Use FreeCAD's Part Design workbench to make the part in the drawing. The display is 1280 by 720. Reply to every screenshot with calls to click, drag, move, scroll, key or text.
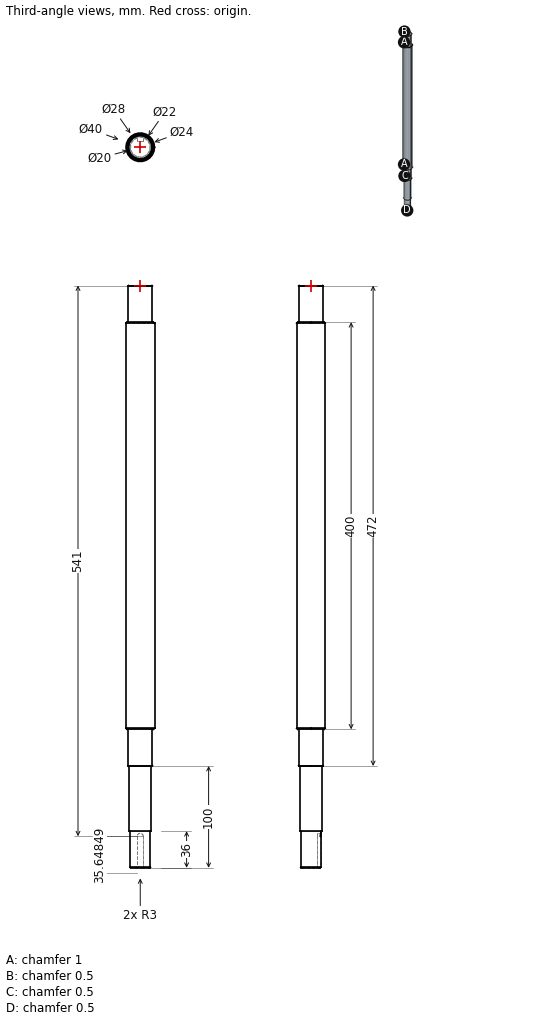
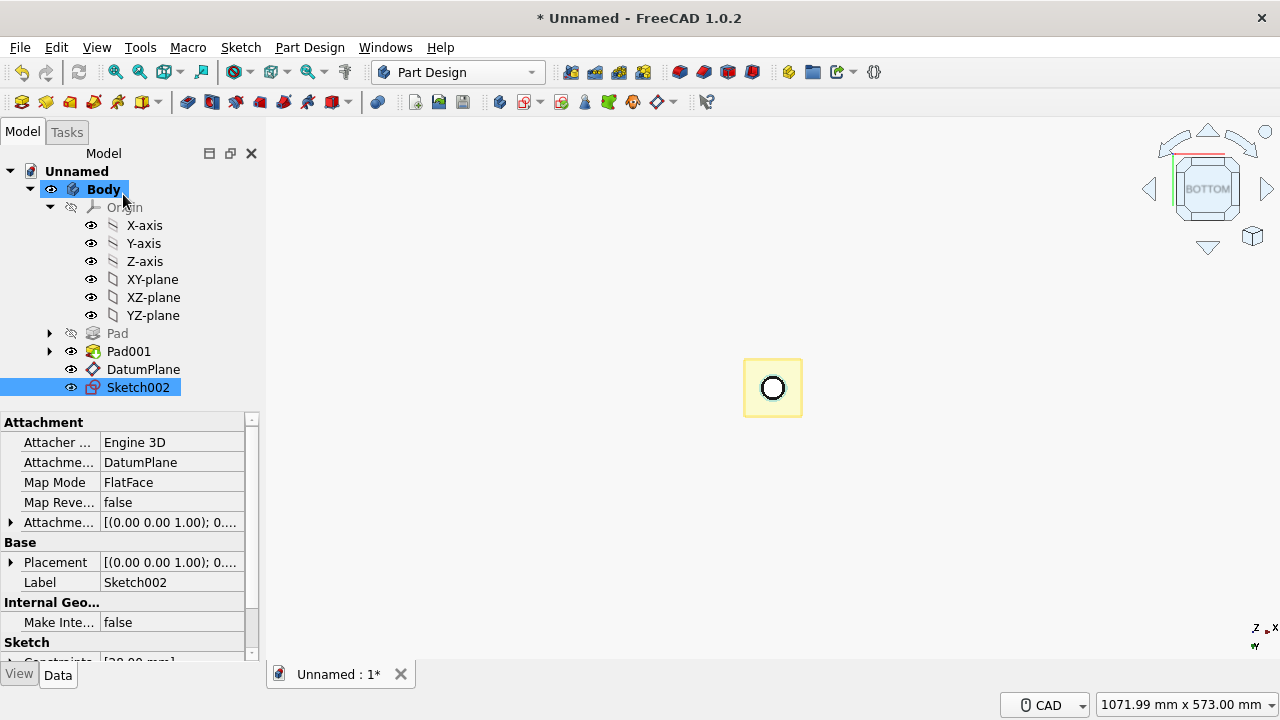
click(22, 102)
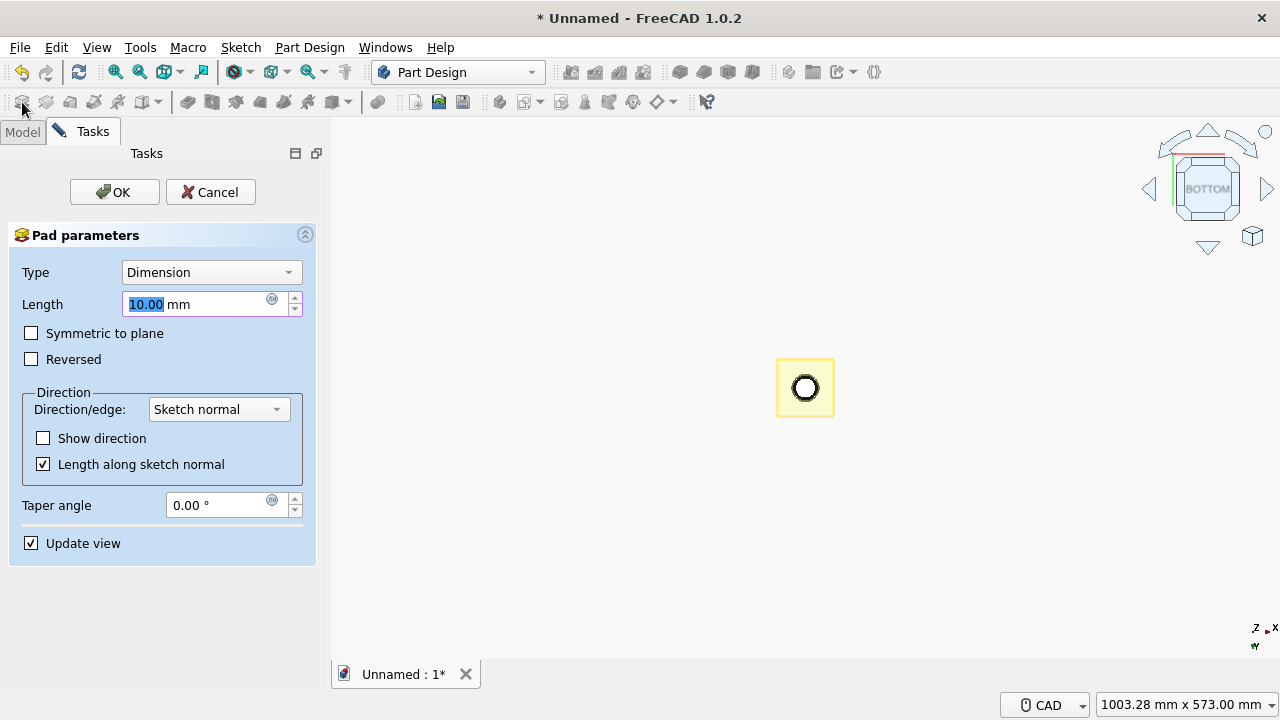
text(400)
key(Tab)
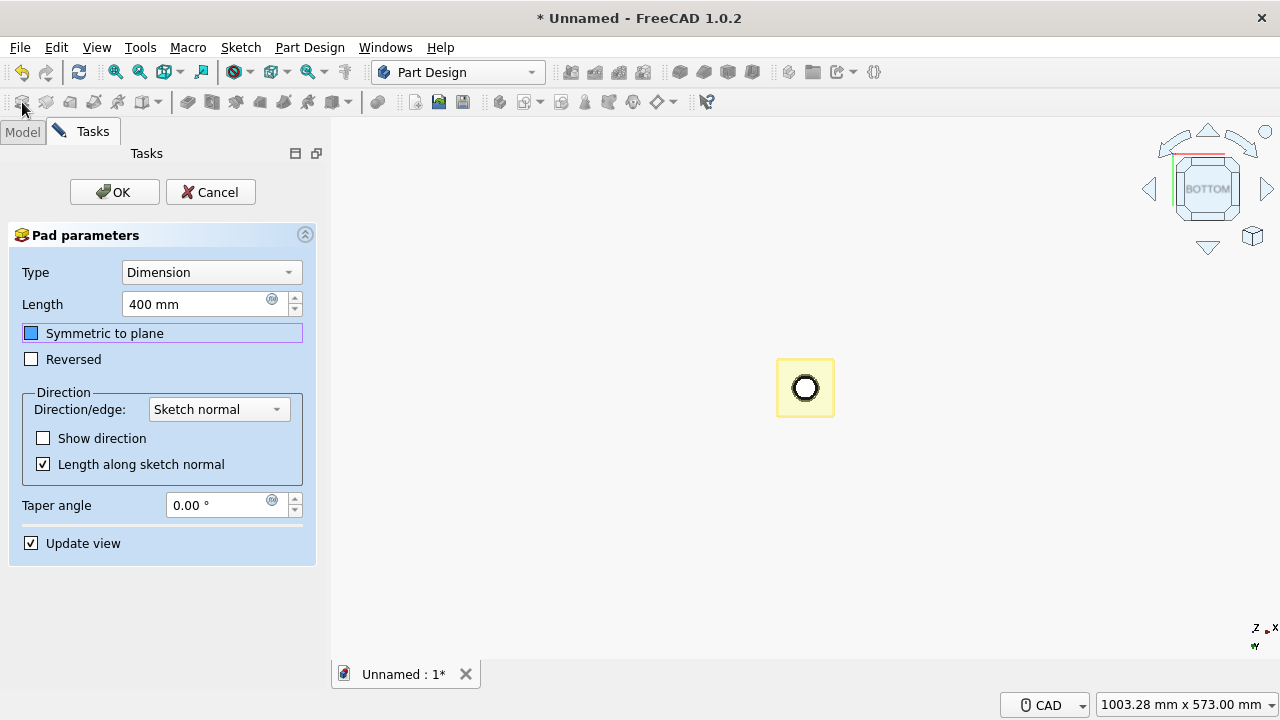
click(30, 359)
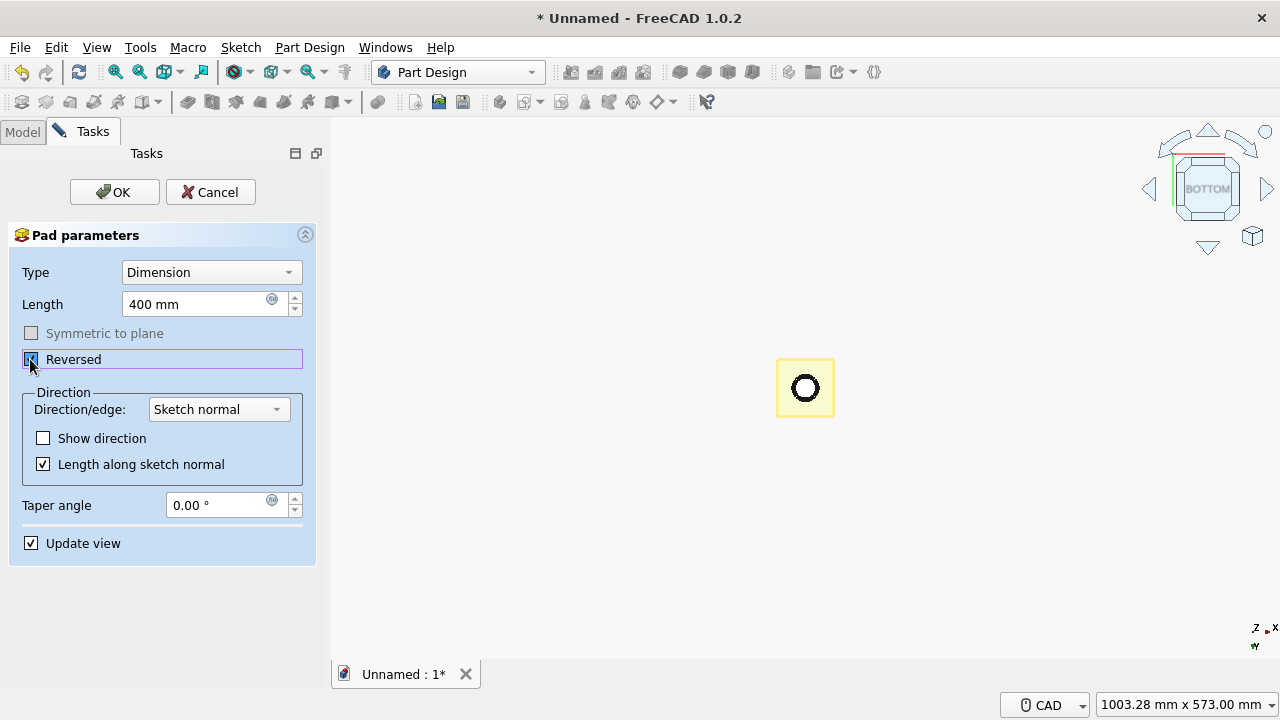
click(115, 192)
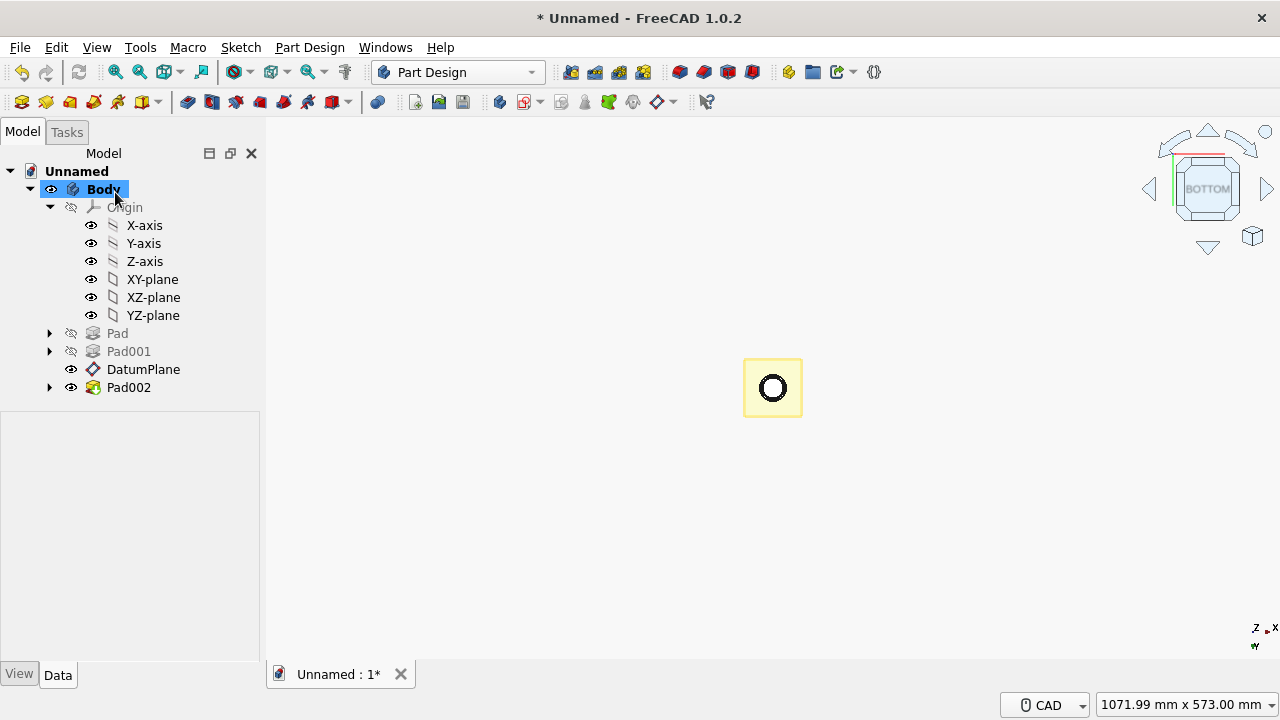
click(116, 369)
key(space)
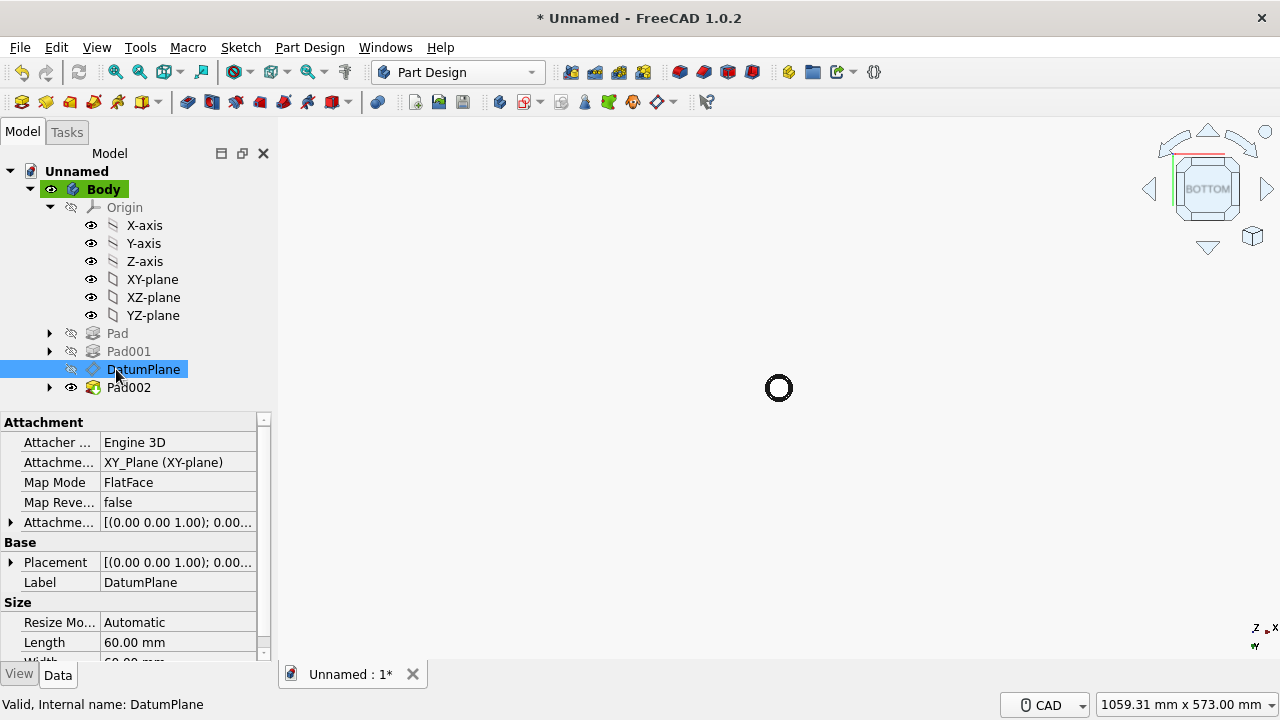
click(116, 72)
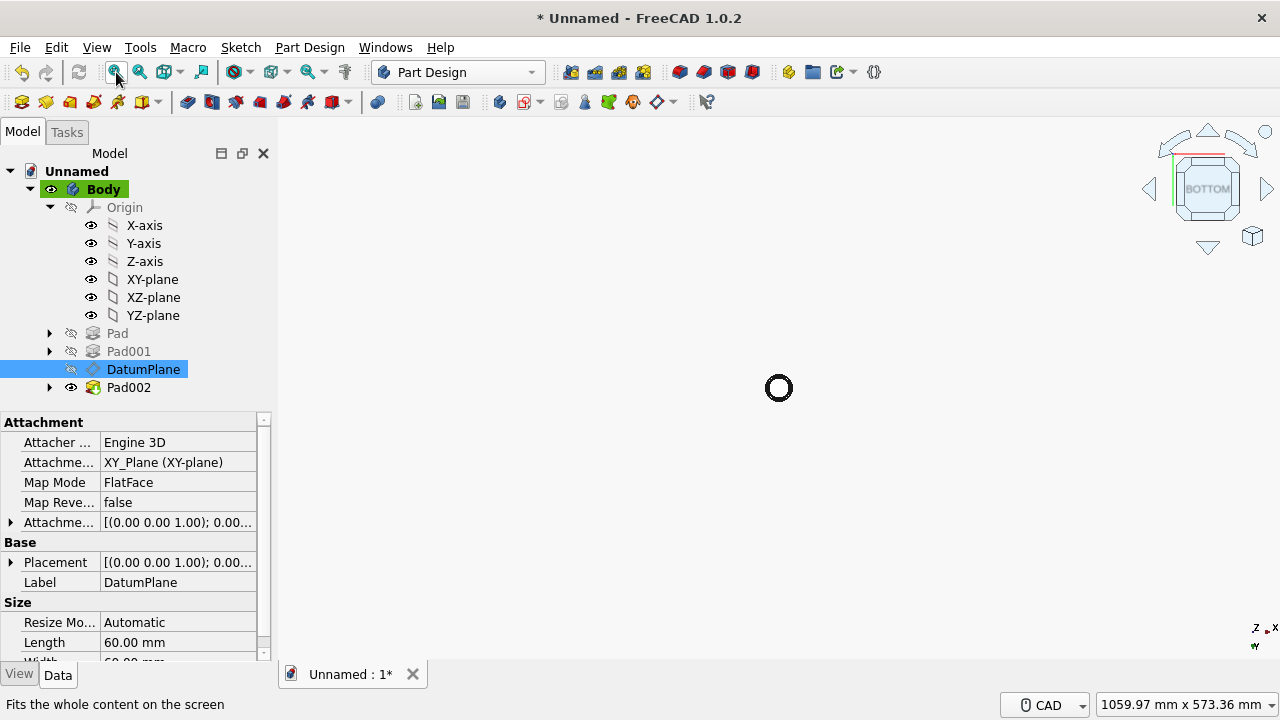
key(0)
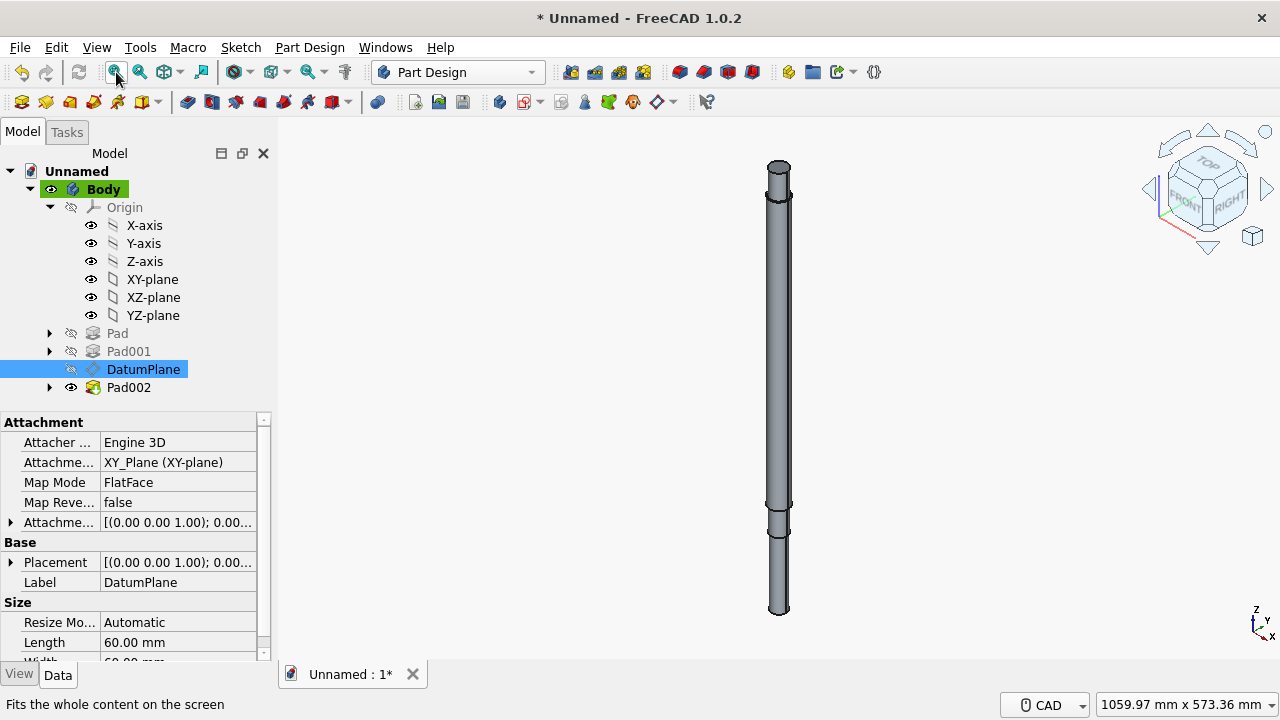
click(767, 198)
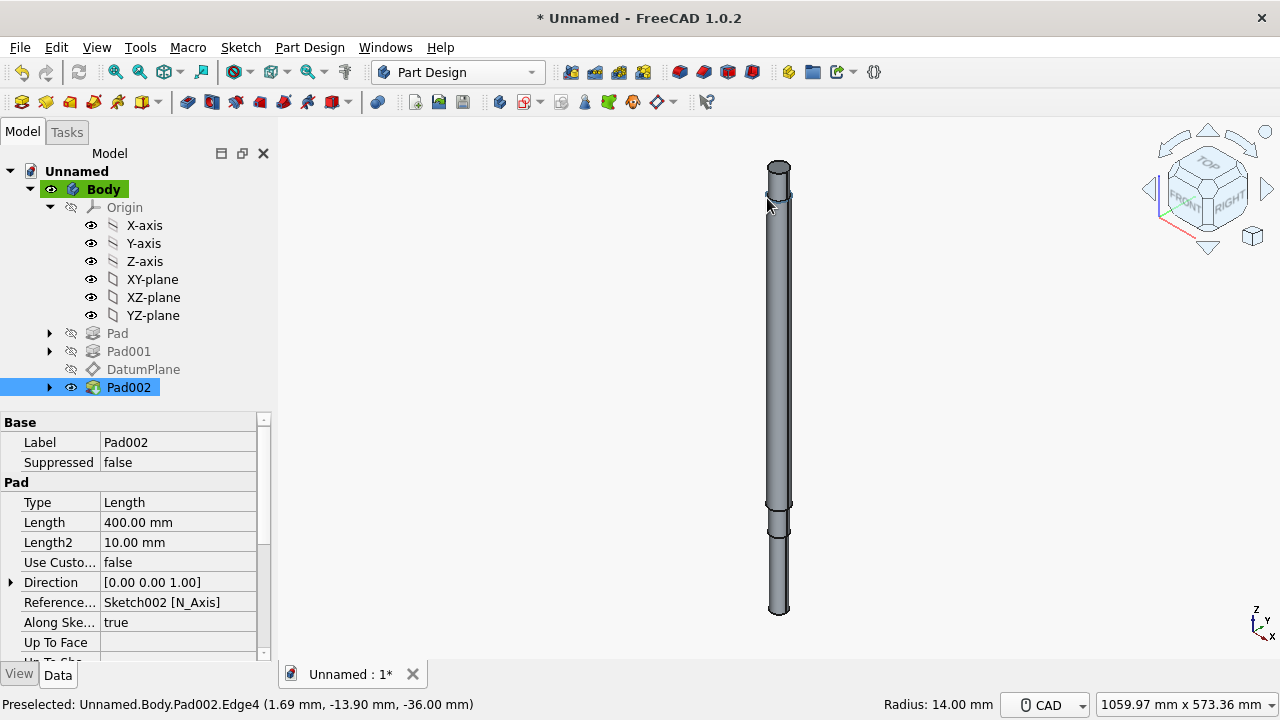
click(773, 510, ctrl)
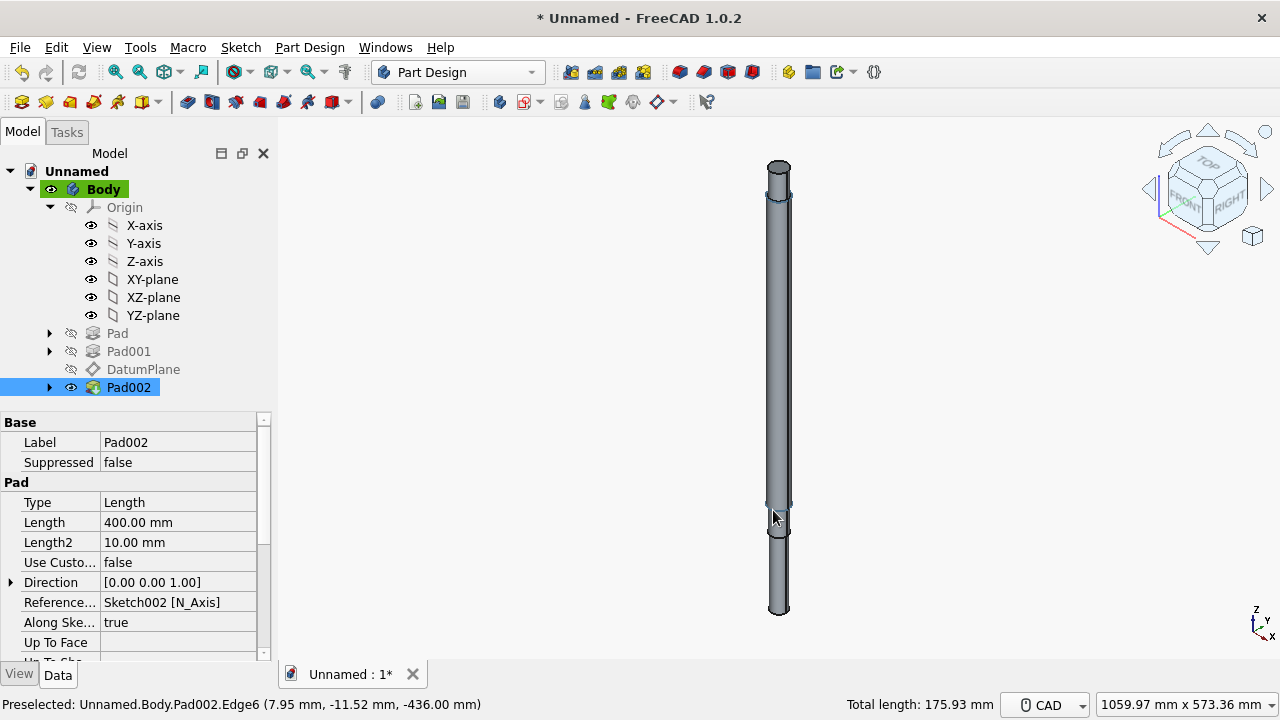
click(704, 72)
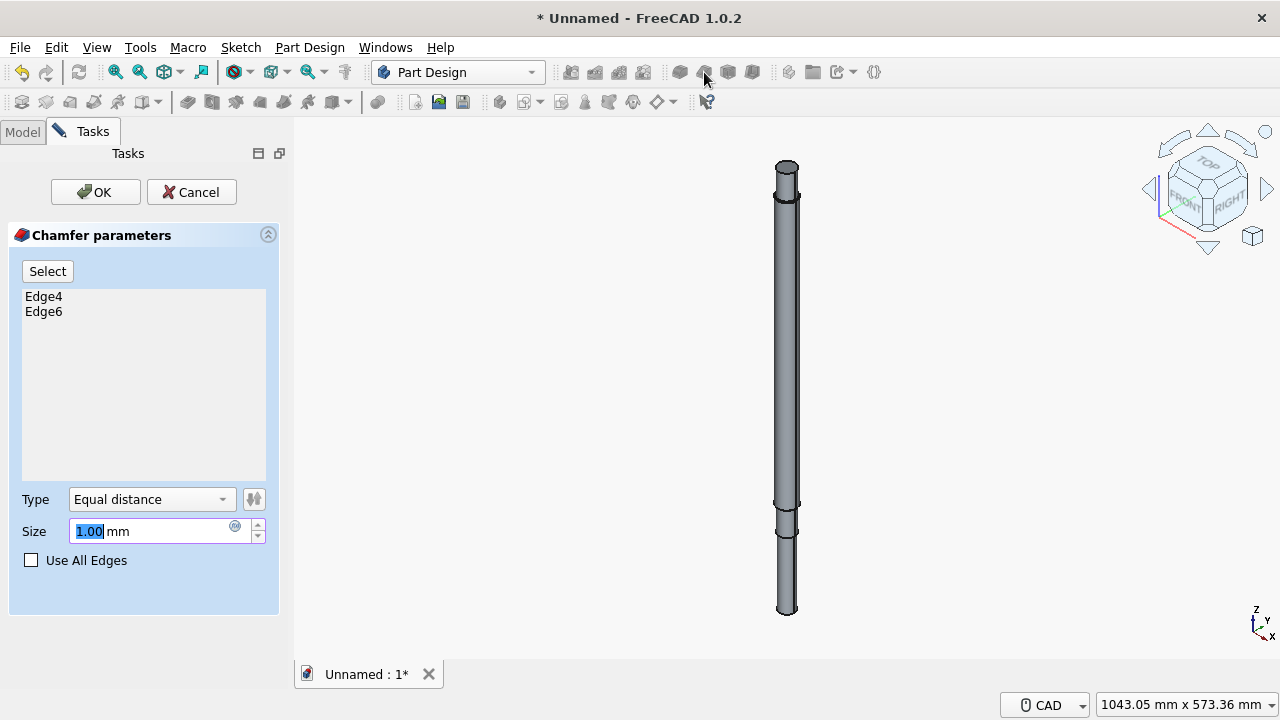
text(1)
key(Tab)